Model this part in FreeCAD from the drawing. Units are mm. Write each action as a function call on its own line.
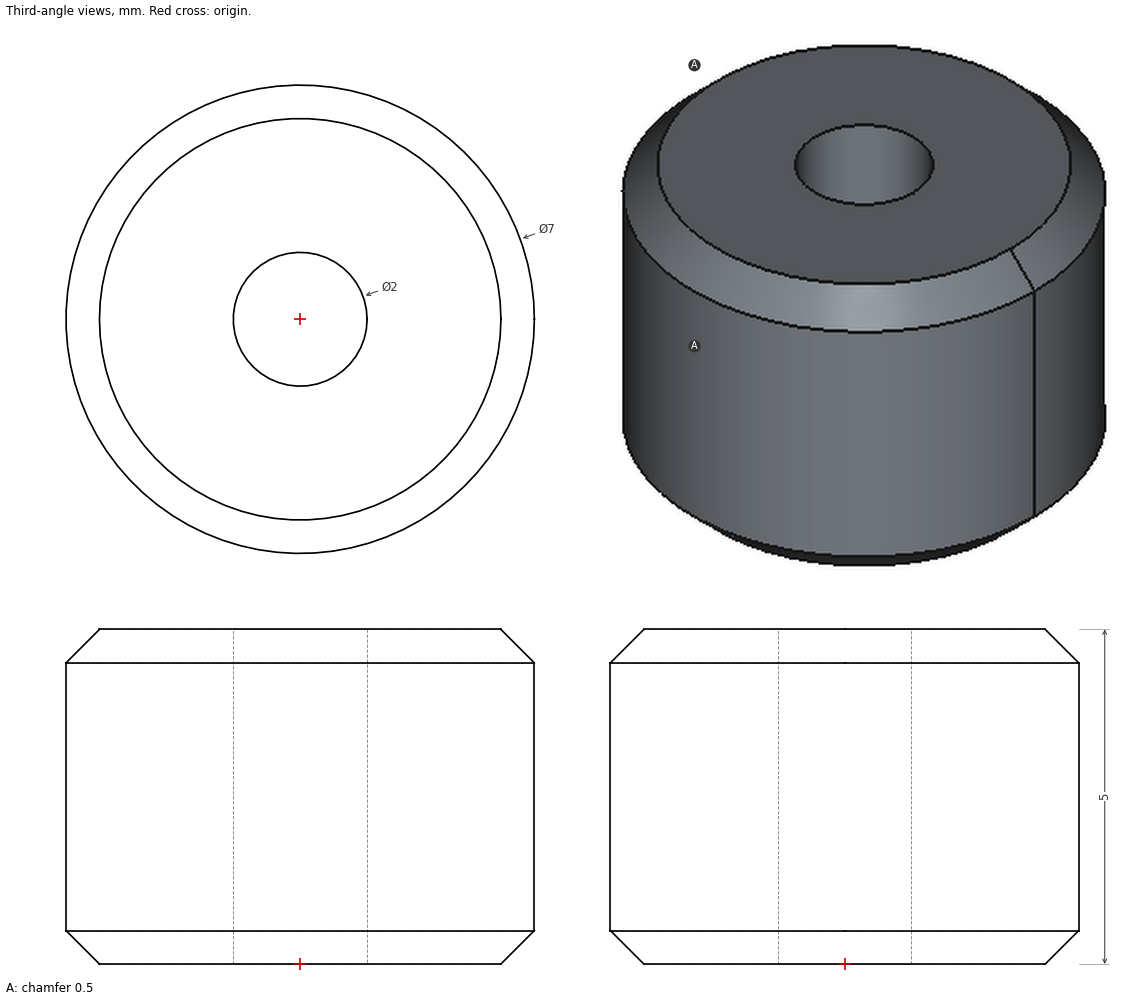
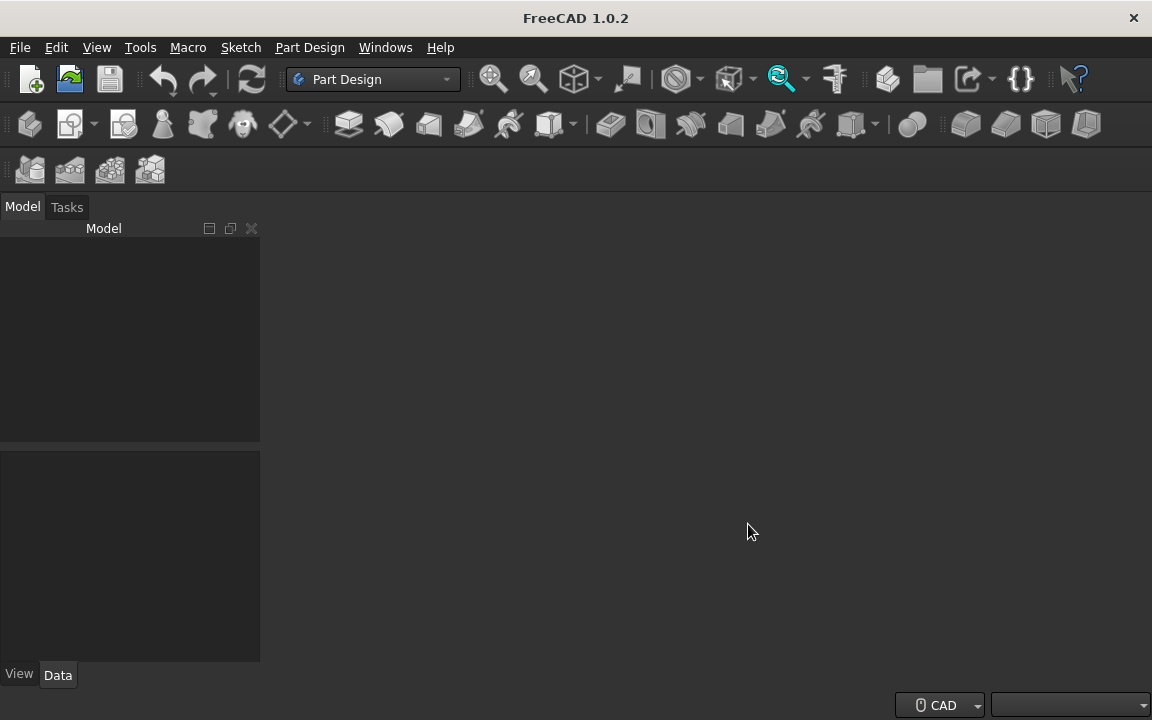
click(30, 80)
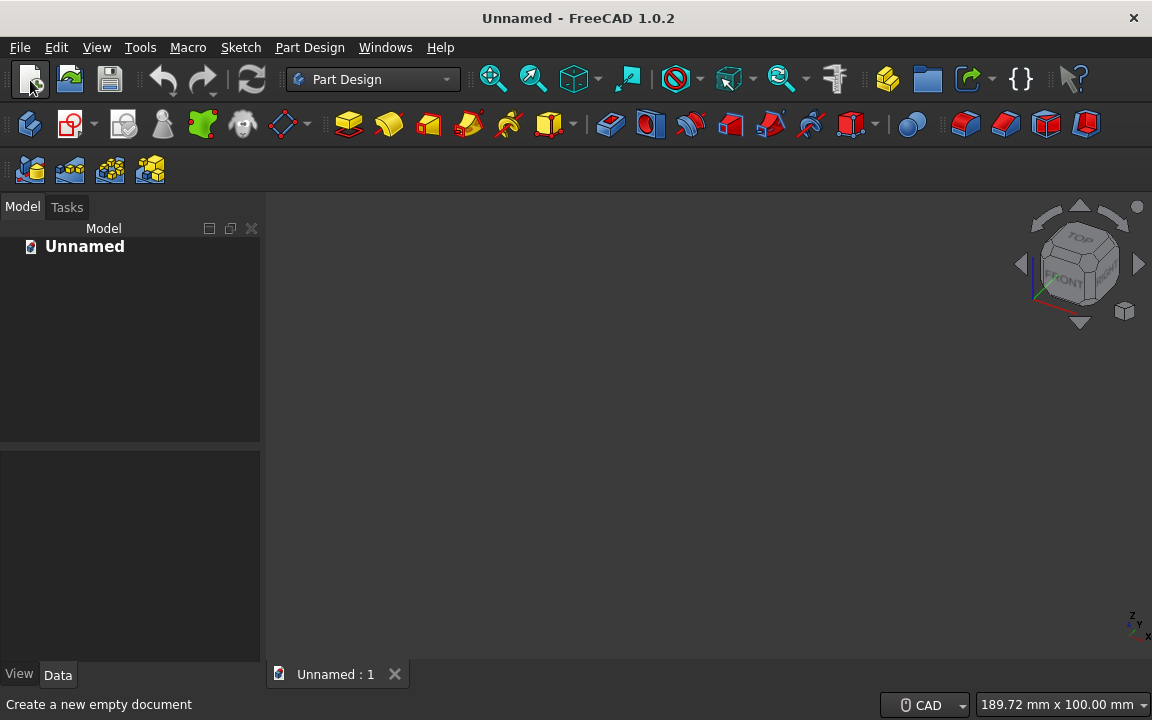
click(70, 124)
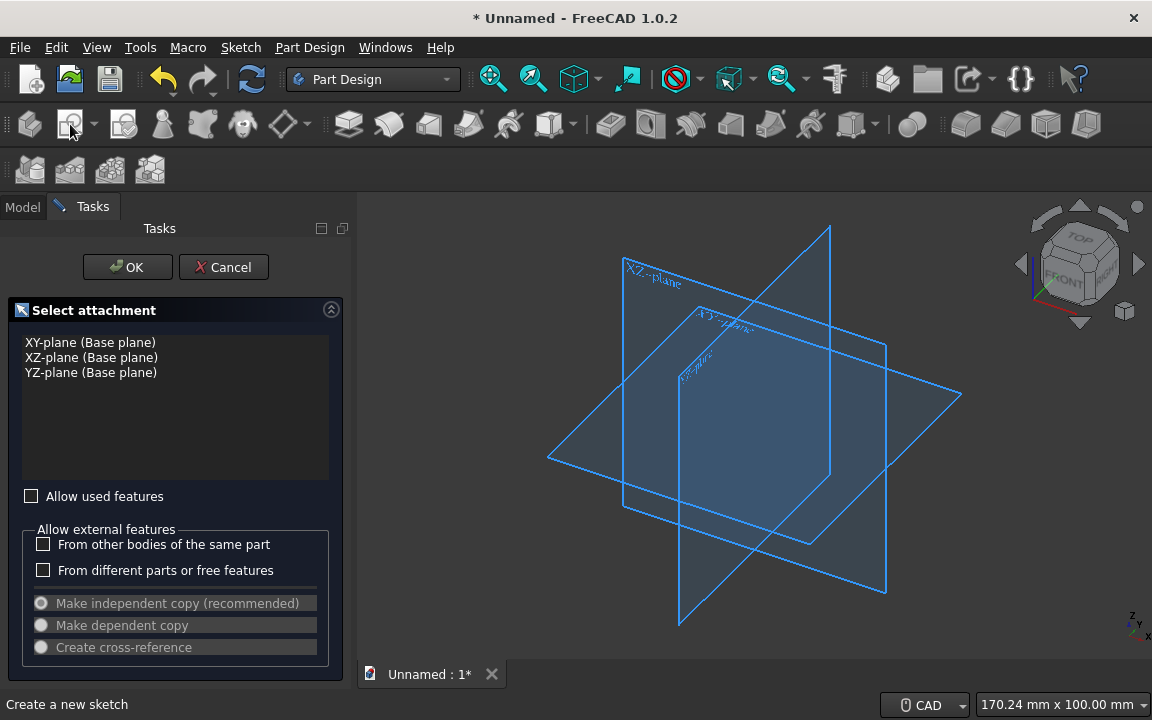
click(82, 342)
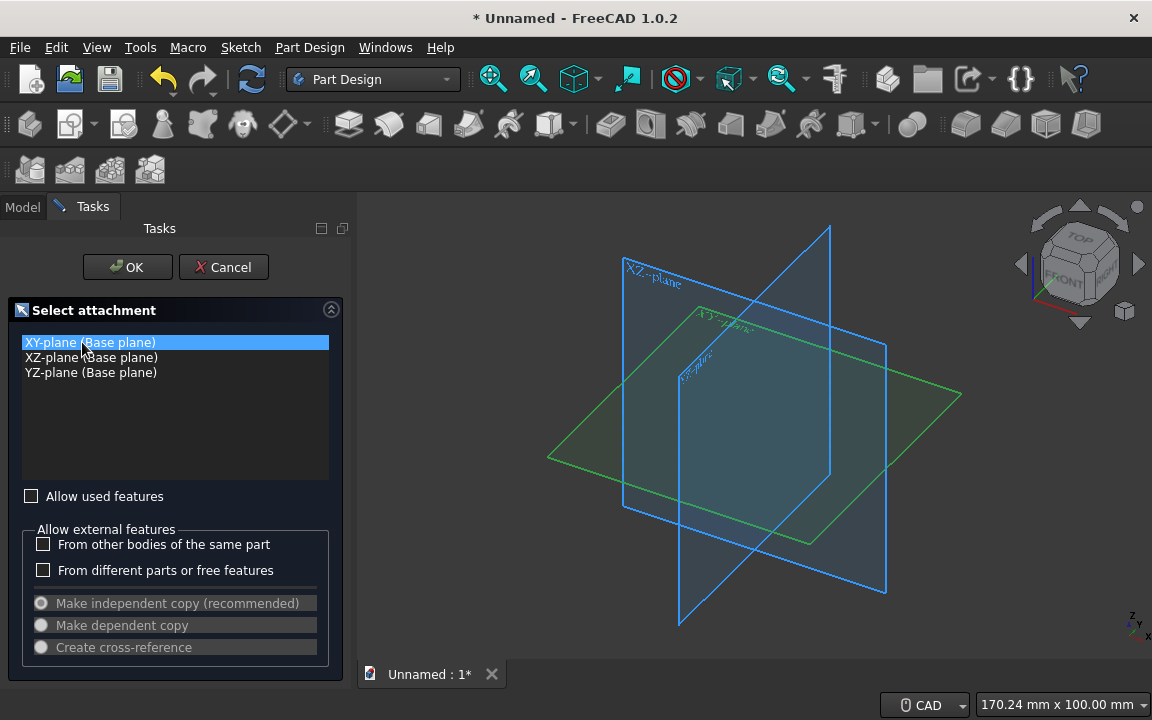
click(128, 267)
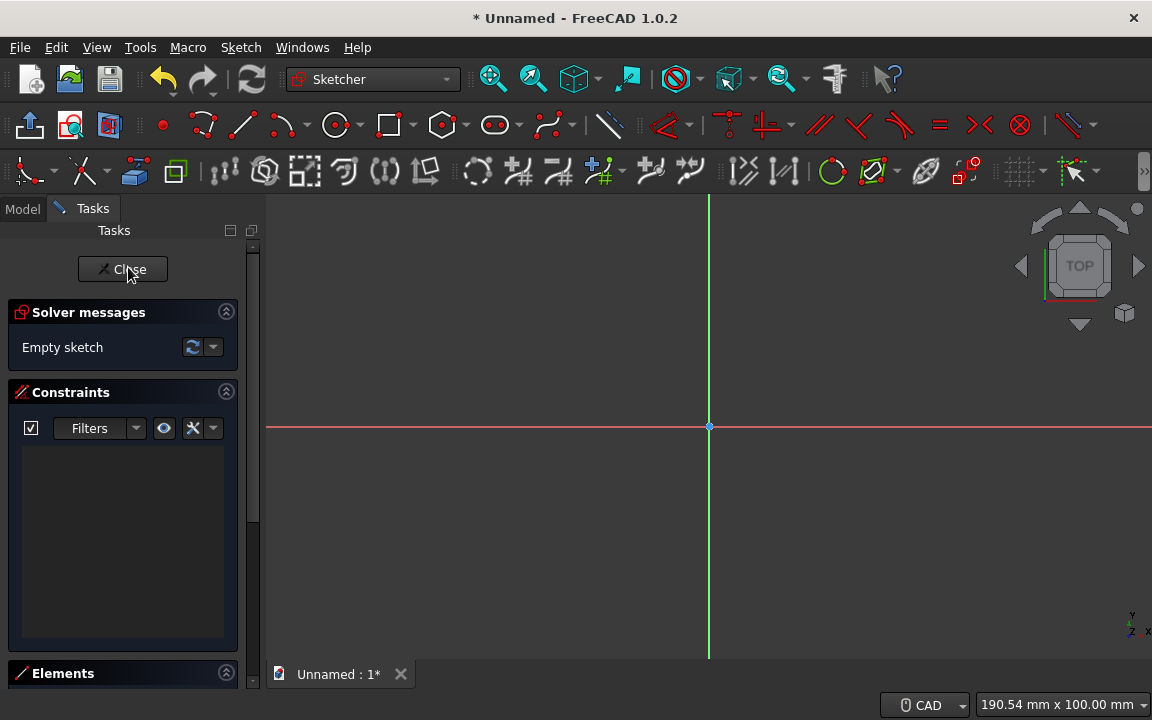
scroll(718, 426, up, 11)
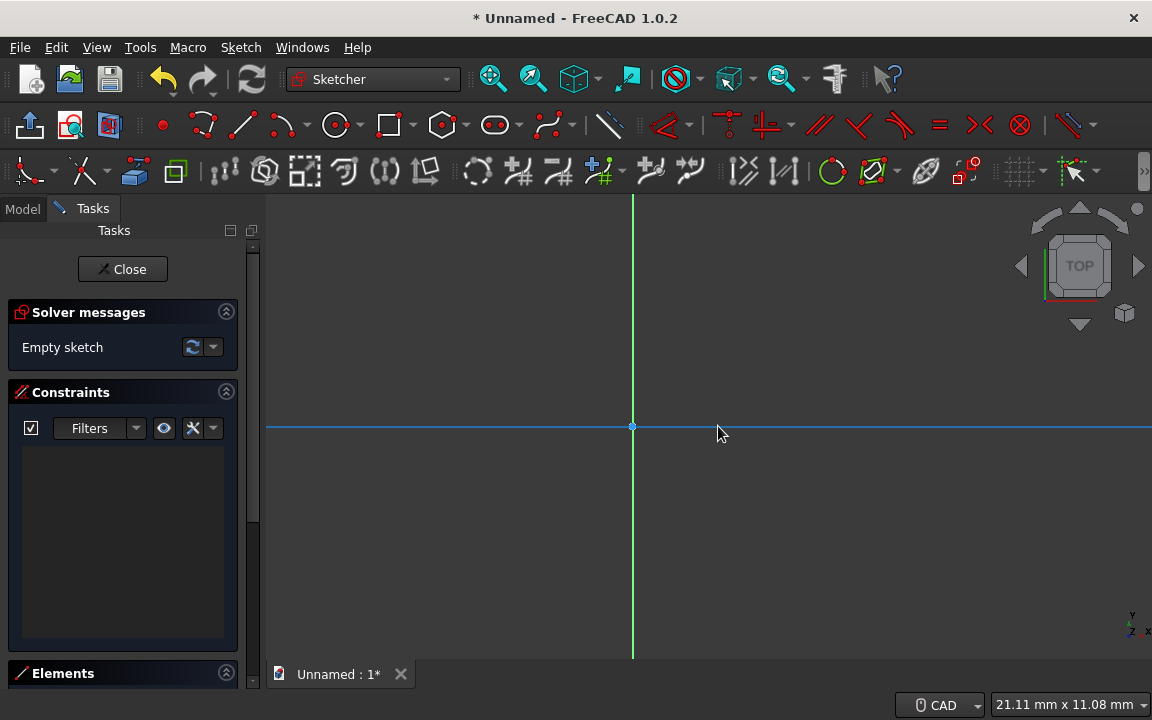
click(336, 126)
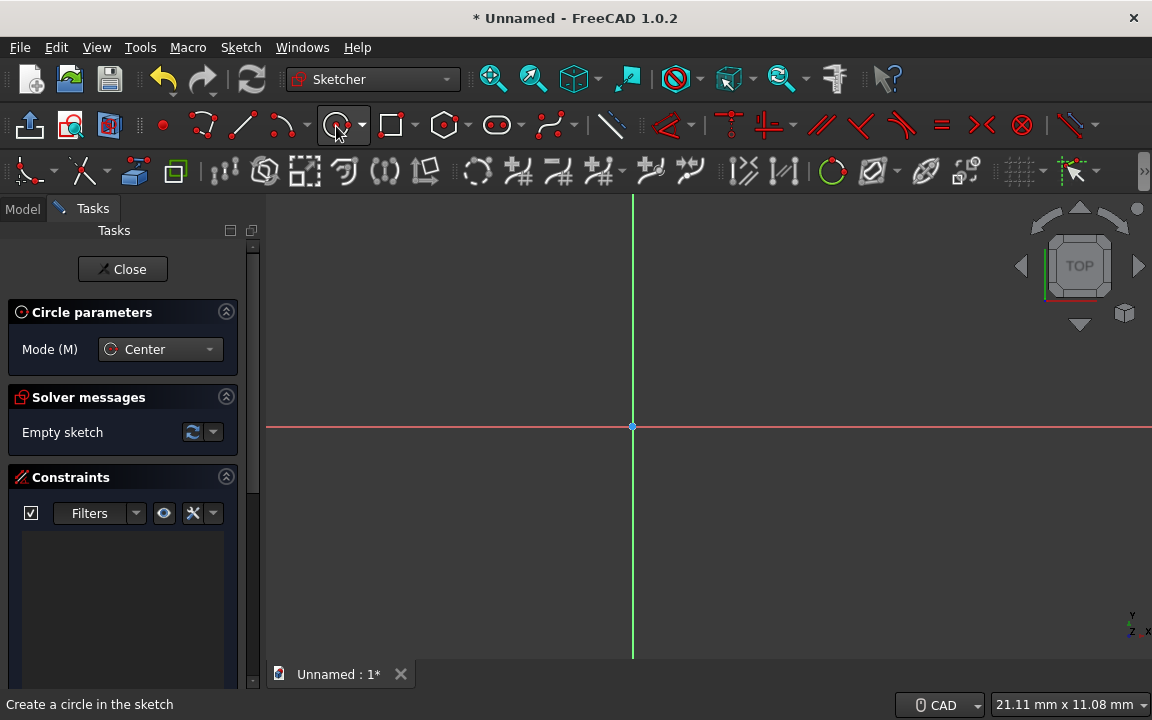
click(633, 426)
click(737, 323)
key(Escape)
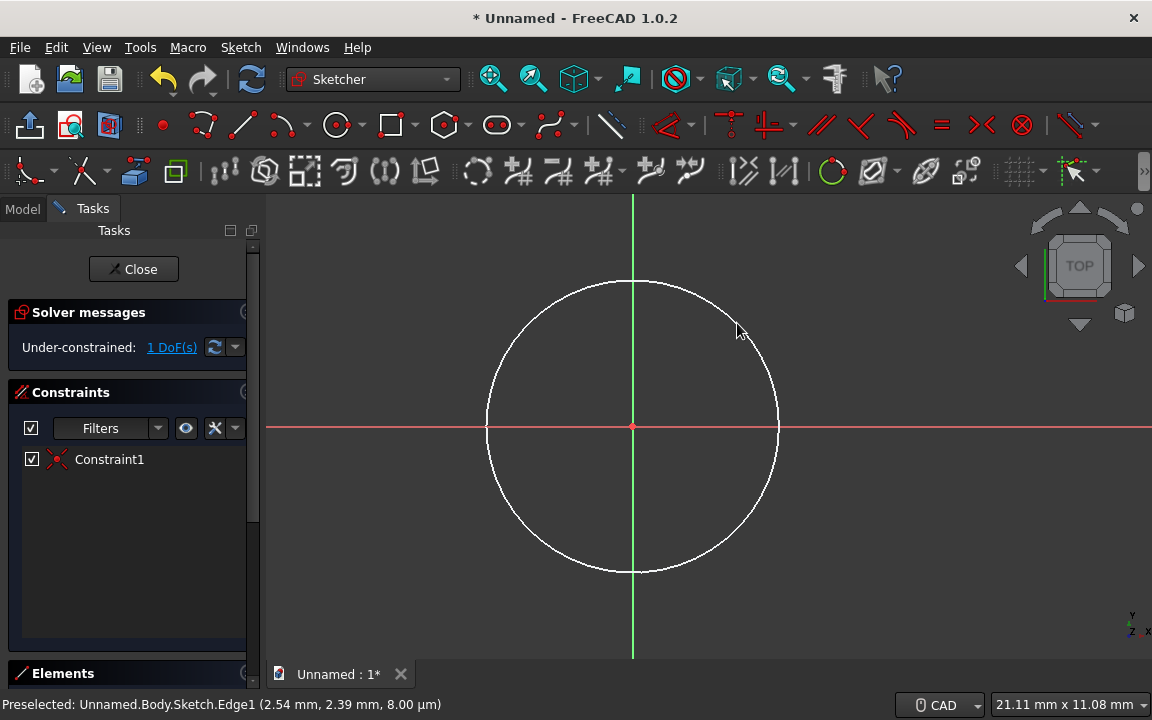
click(666, 126)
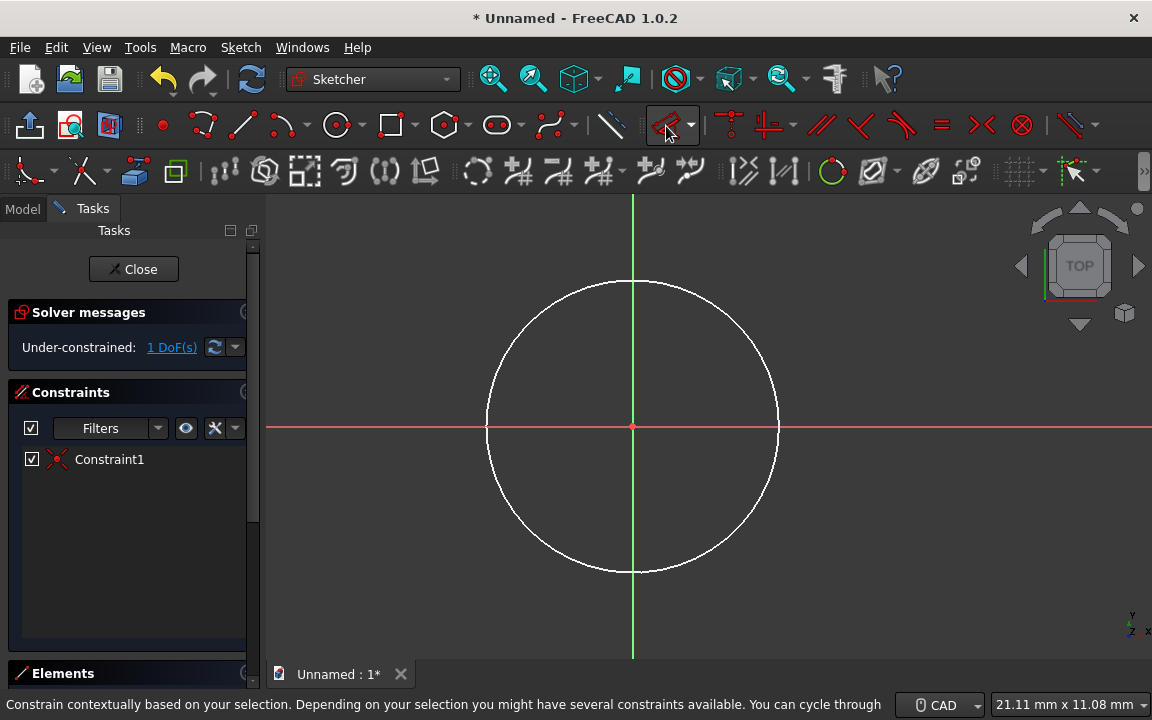
click(736, 323)
click(759, 300)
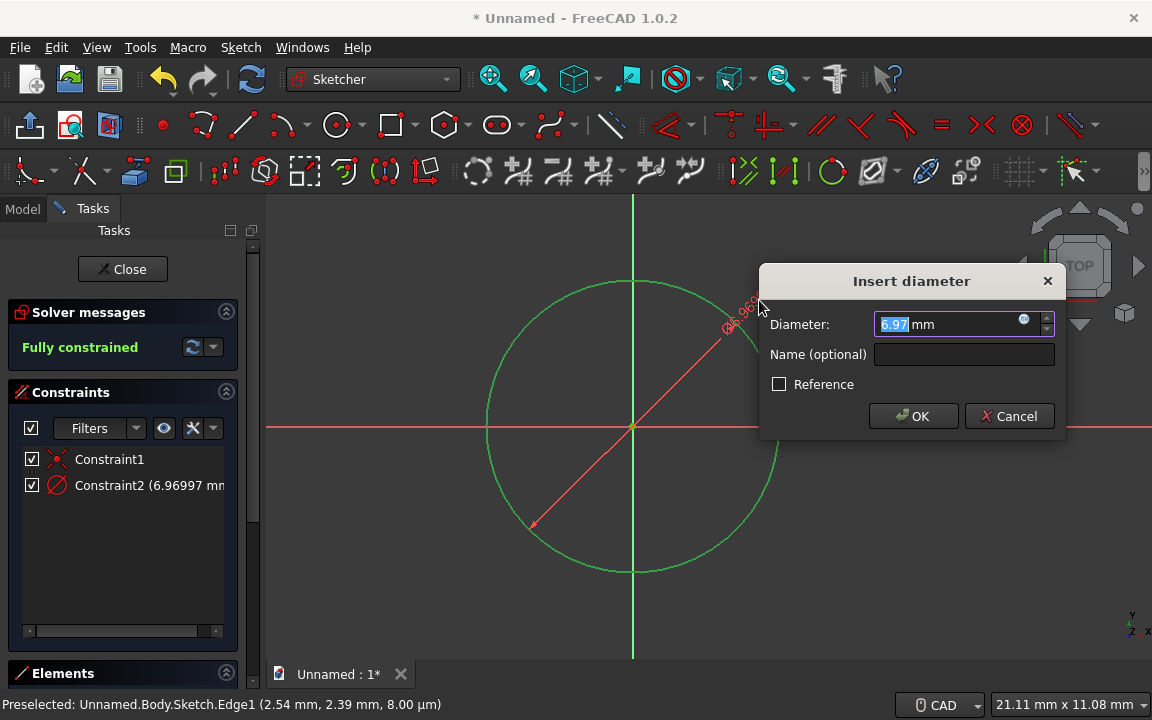
text(7)
key(Return)
key(Escape)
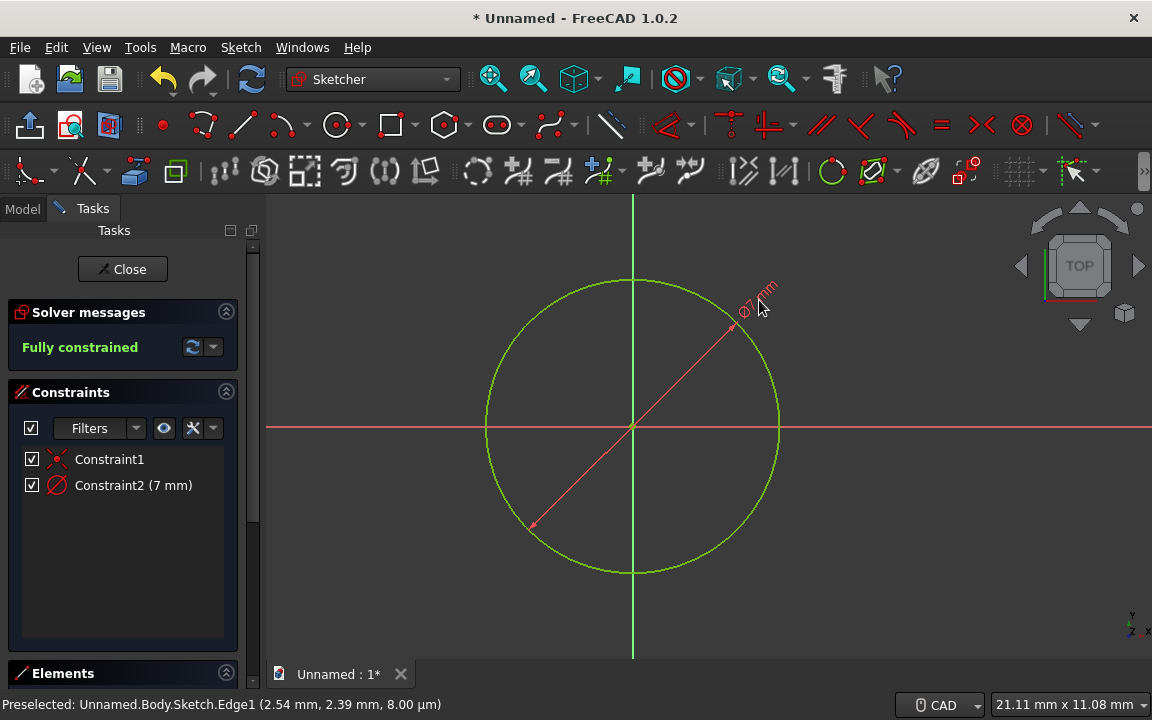
click(123, 269)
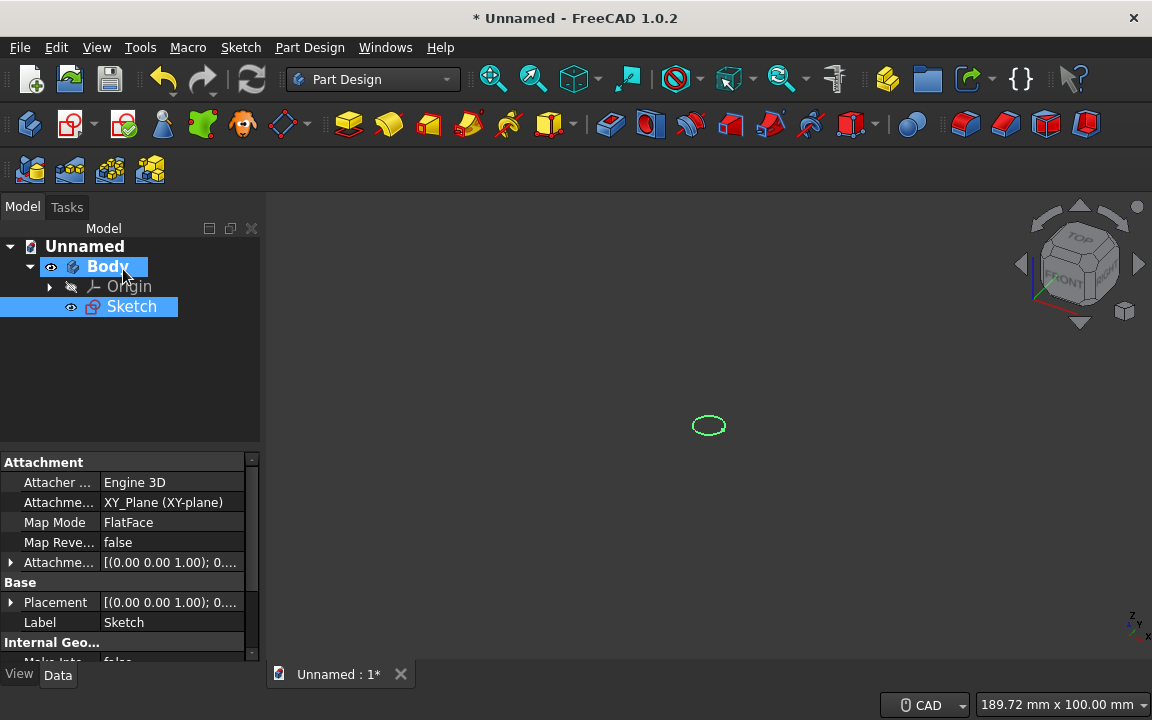
click(350, 124)